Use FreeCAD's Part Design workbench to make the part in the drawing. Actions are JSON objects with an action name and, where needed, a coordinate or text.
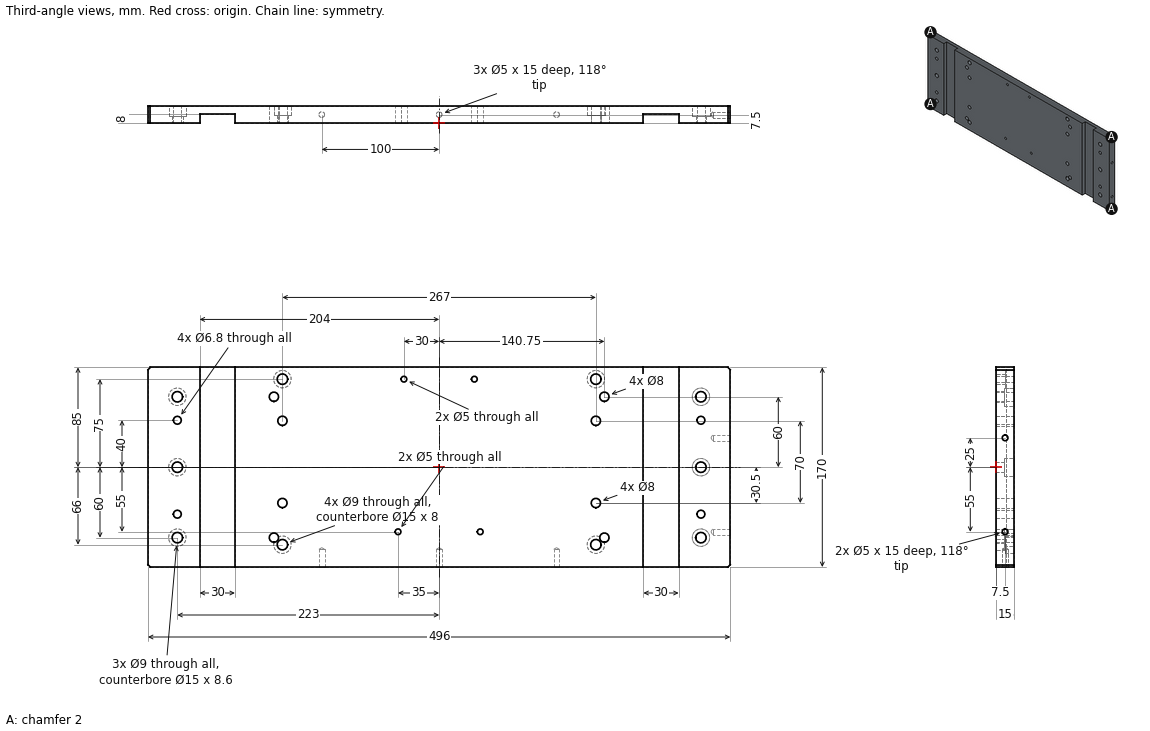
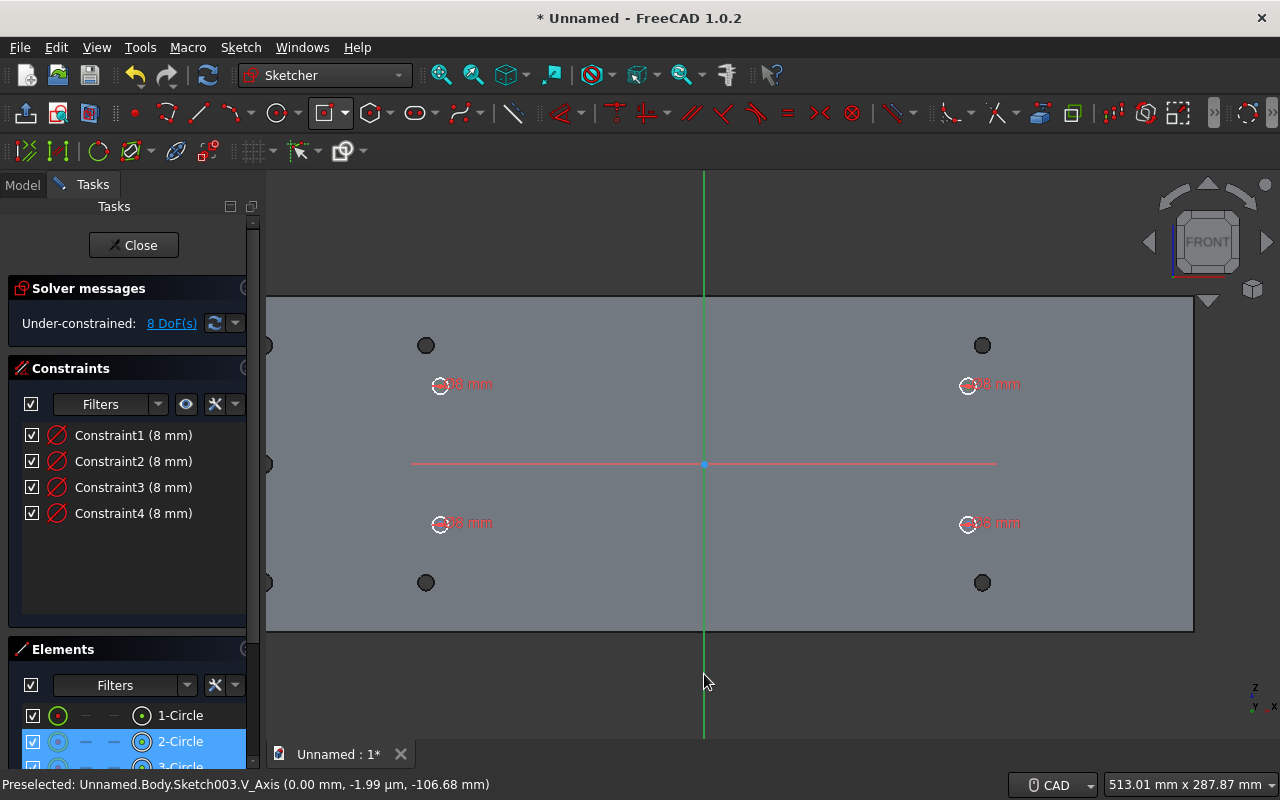
{"action": "left_click", "coordinate": [820, 114]}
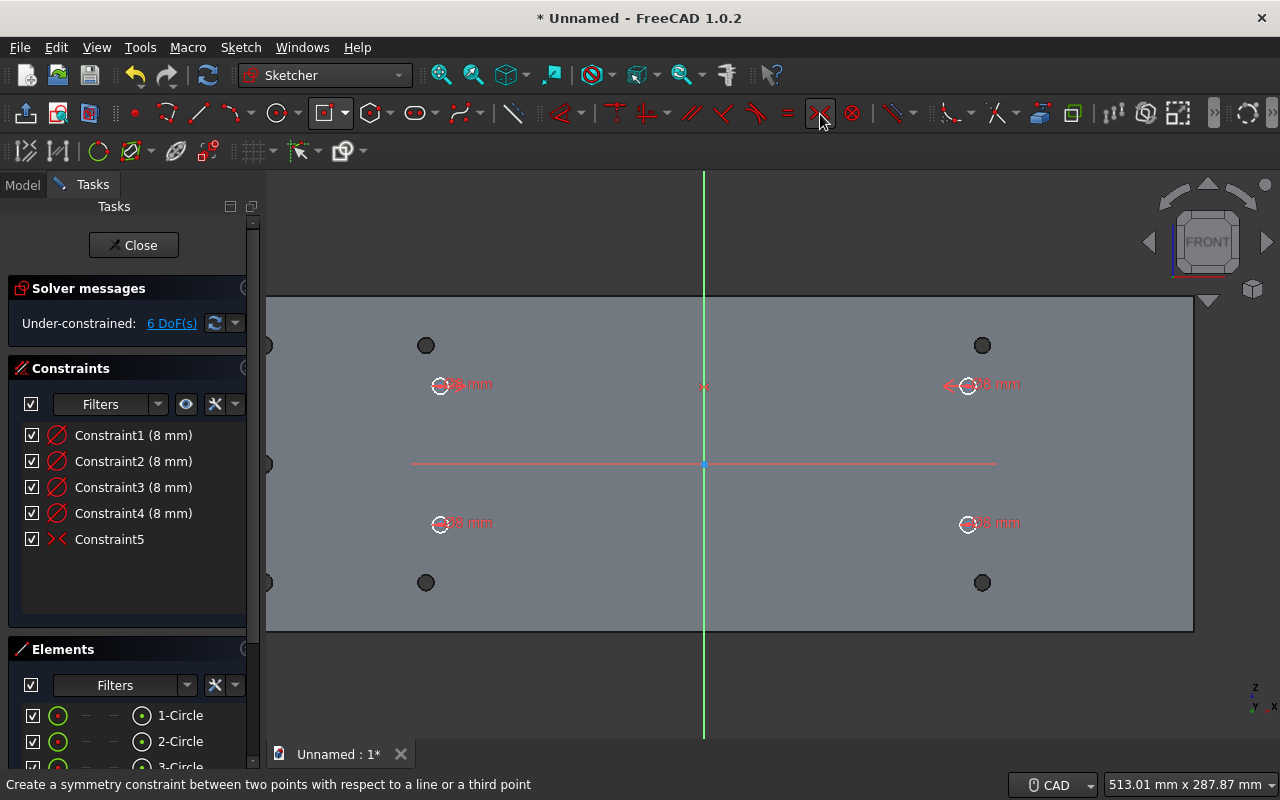
{"action": "left_click", "coordinate": [968, 525]}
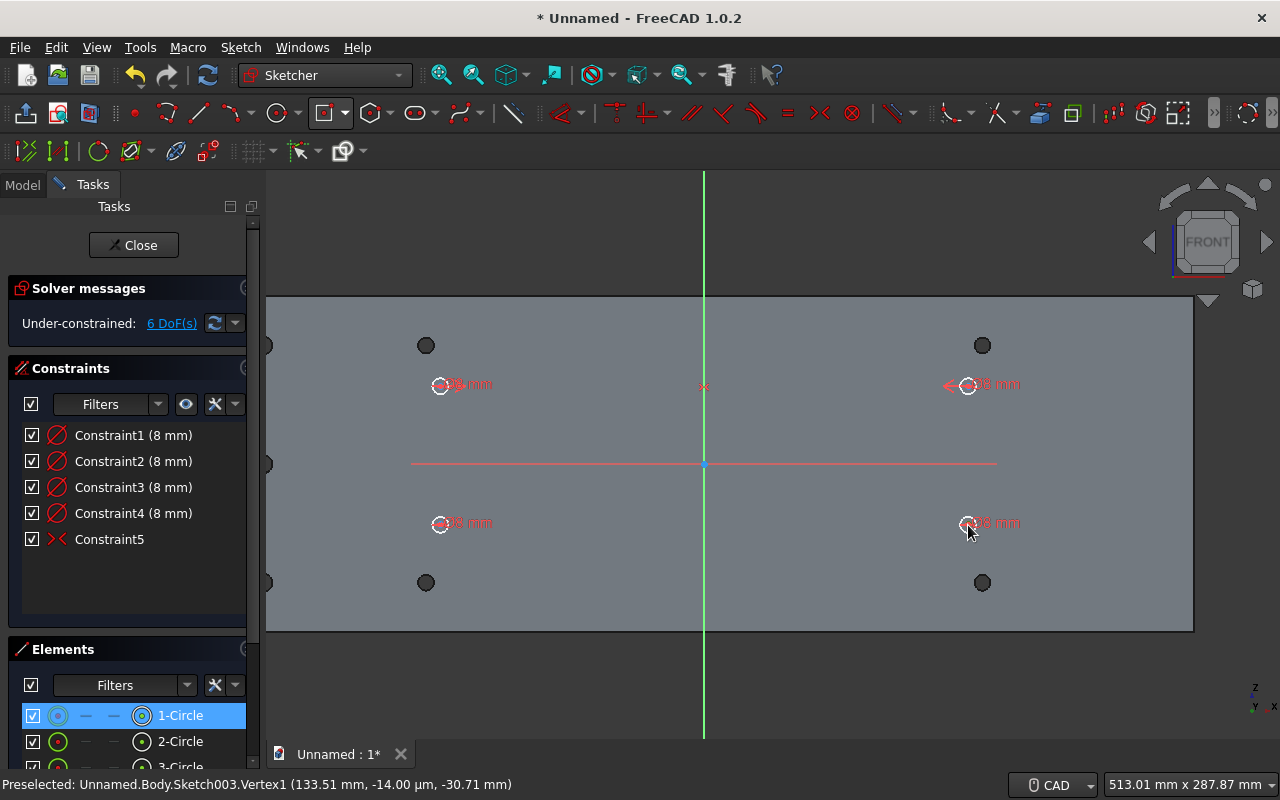
{"action": "left_click", "coordinate": [440, 525]}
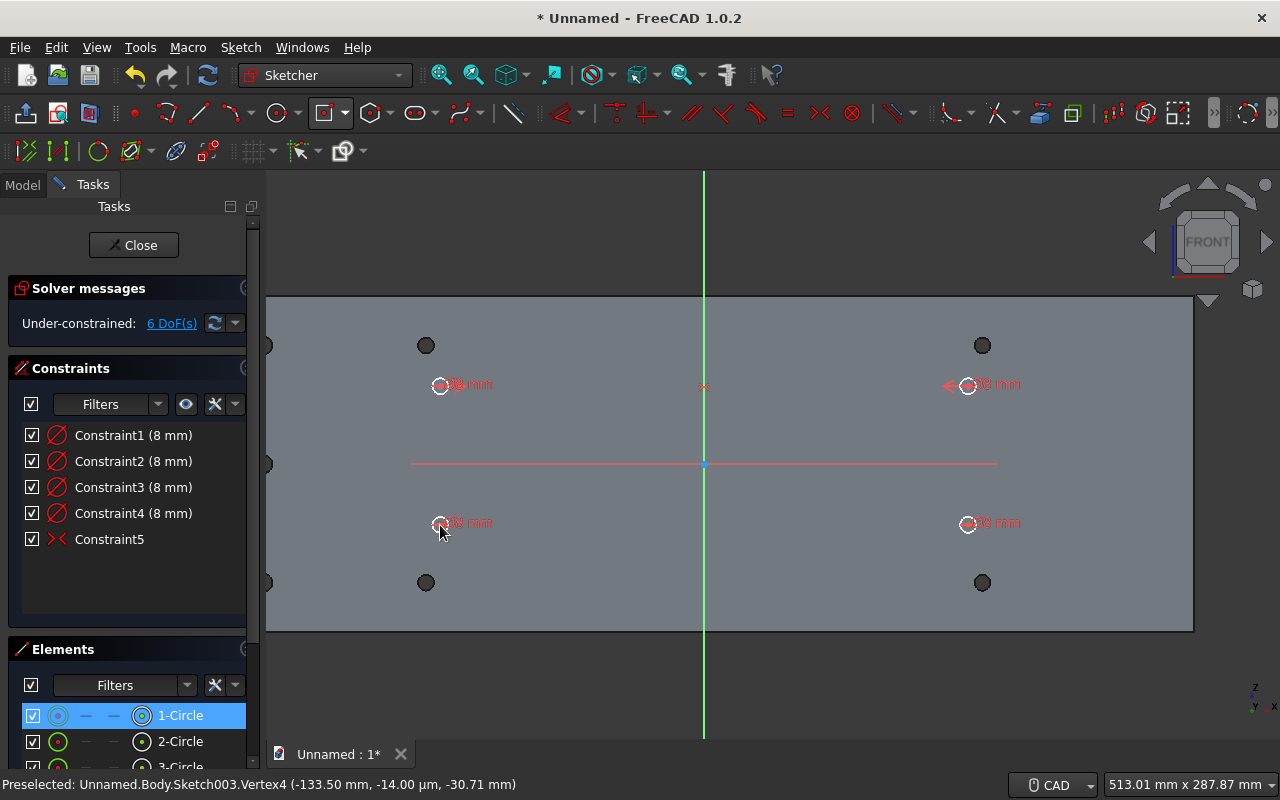
{"action": "left_click", "coordinate": [704, 674]}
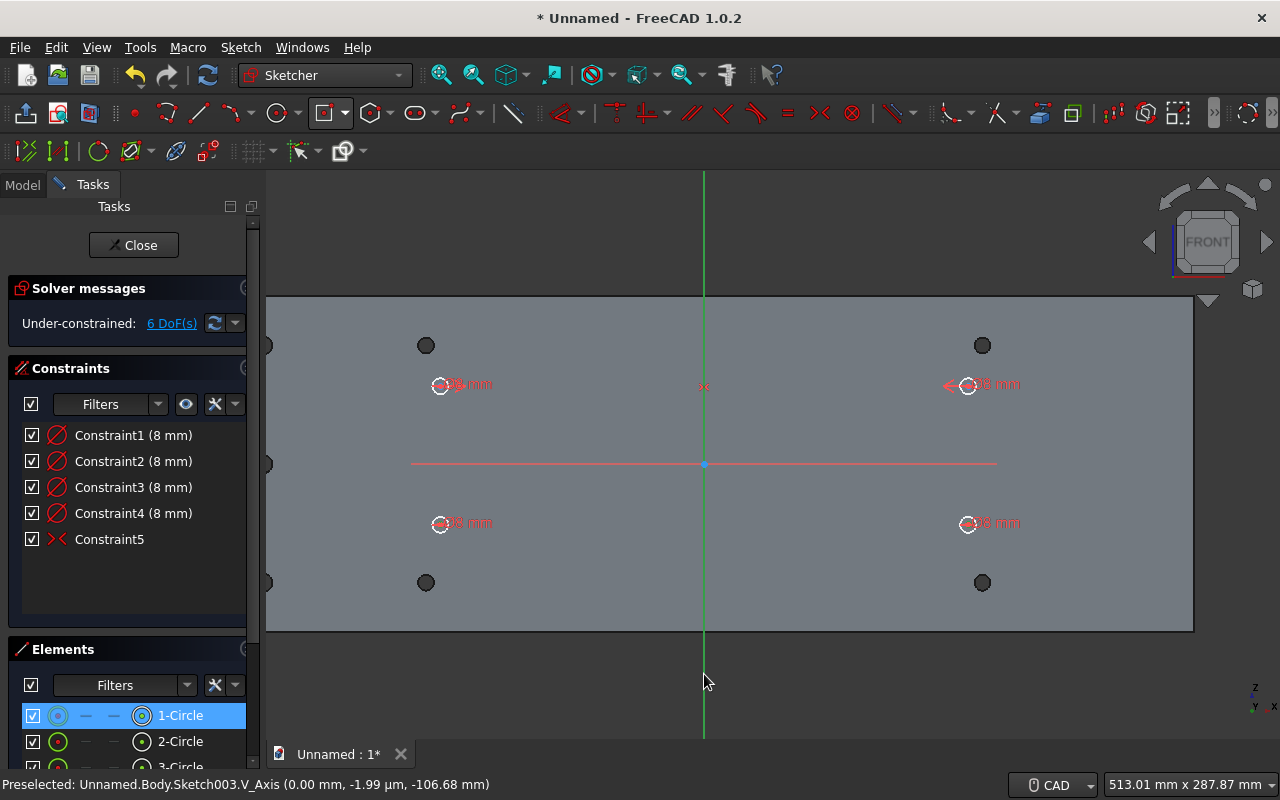
{"action": "left_click", "coordinate": [820, 114]}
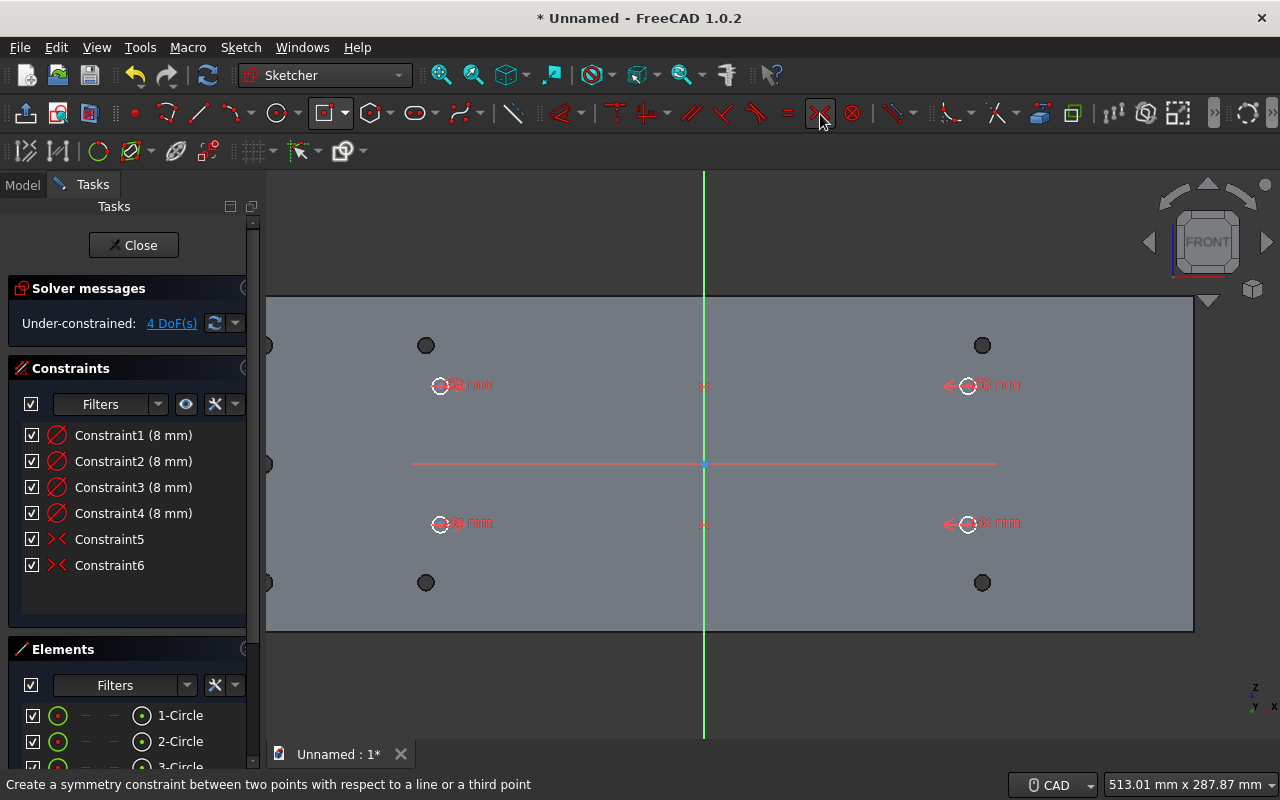
{"action": "left_click", "coordinate": [560, 114]}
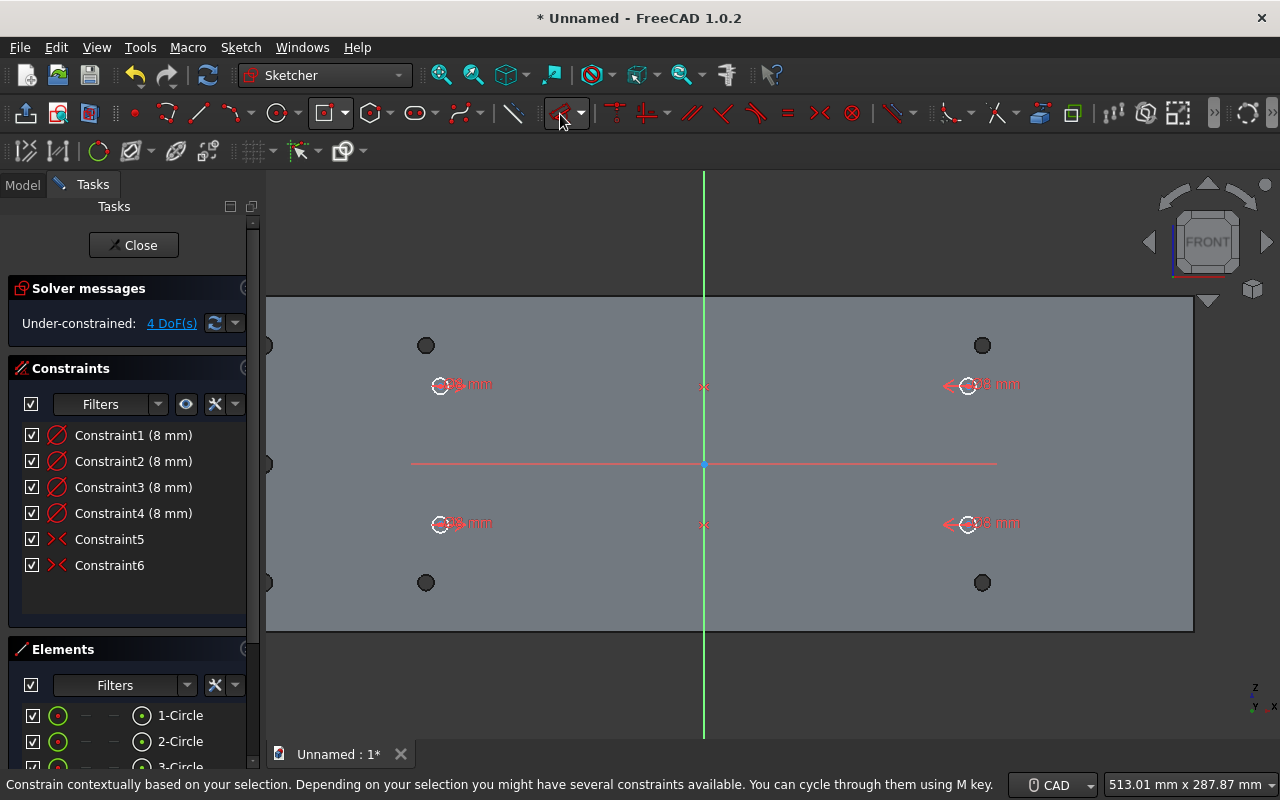
{"action": "left_click", "coordinate": [968, 525]}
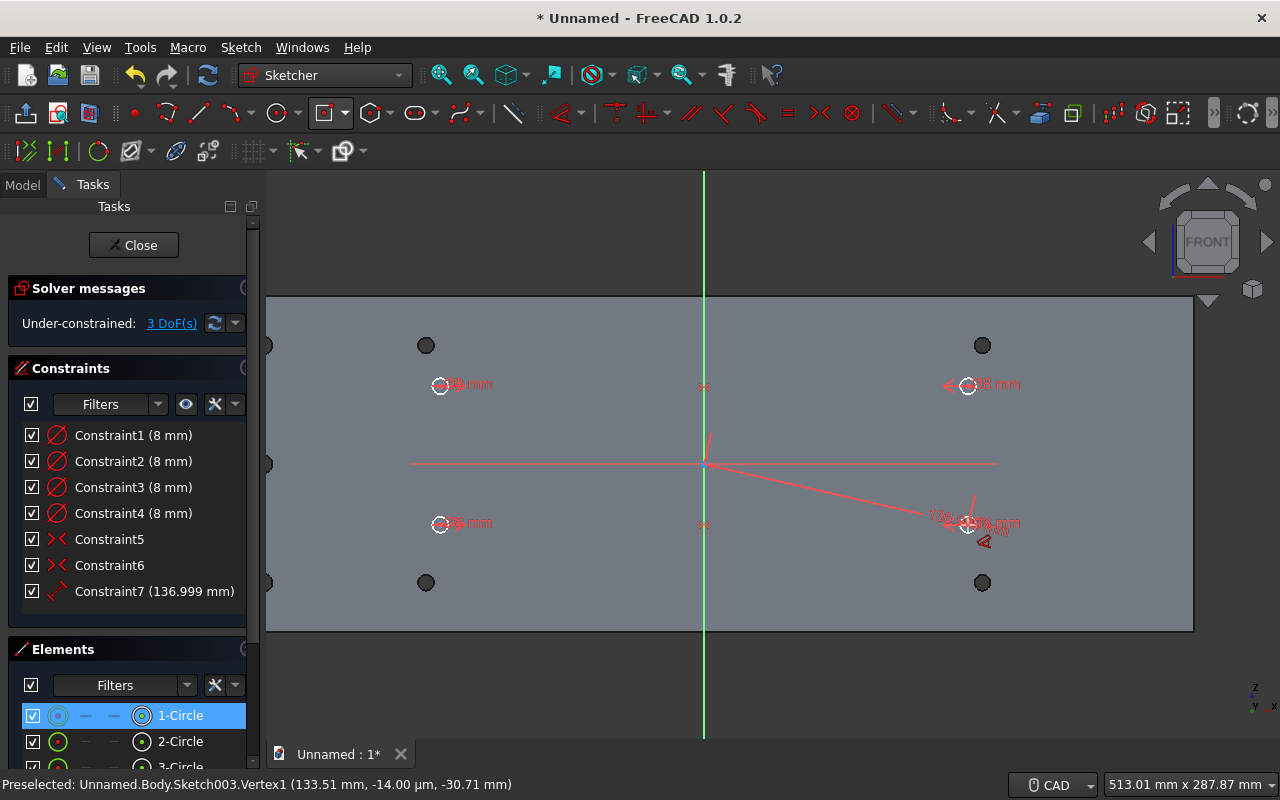
{"action": "left_click", "coordinate": [968, 386]}
{"action": "left_click", "coordinate": [1002, 424]}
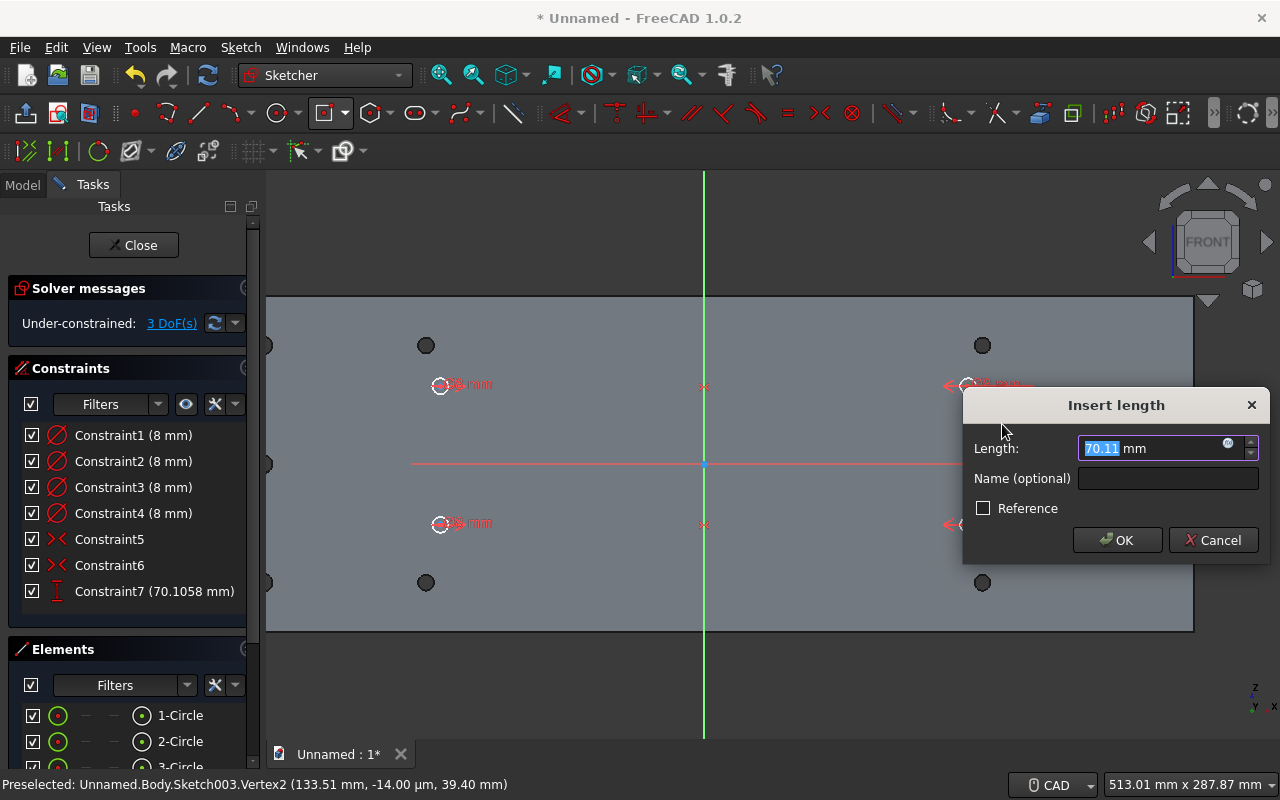
{"action": "type", "text": "70"}
{"action": "key", "text": "Return"}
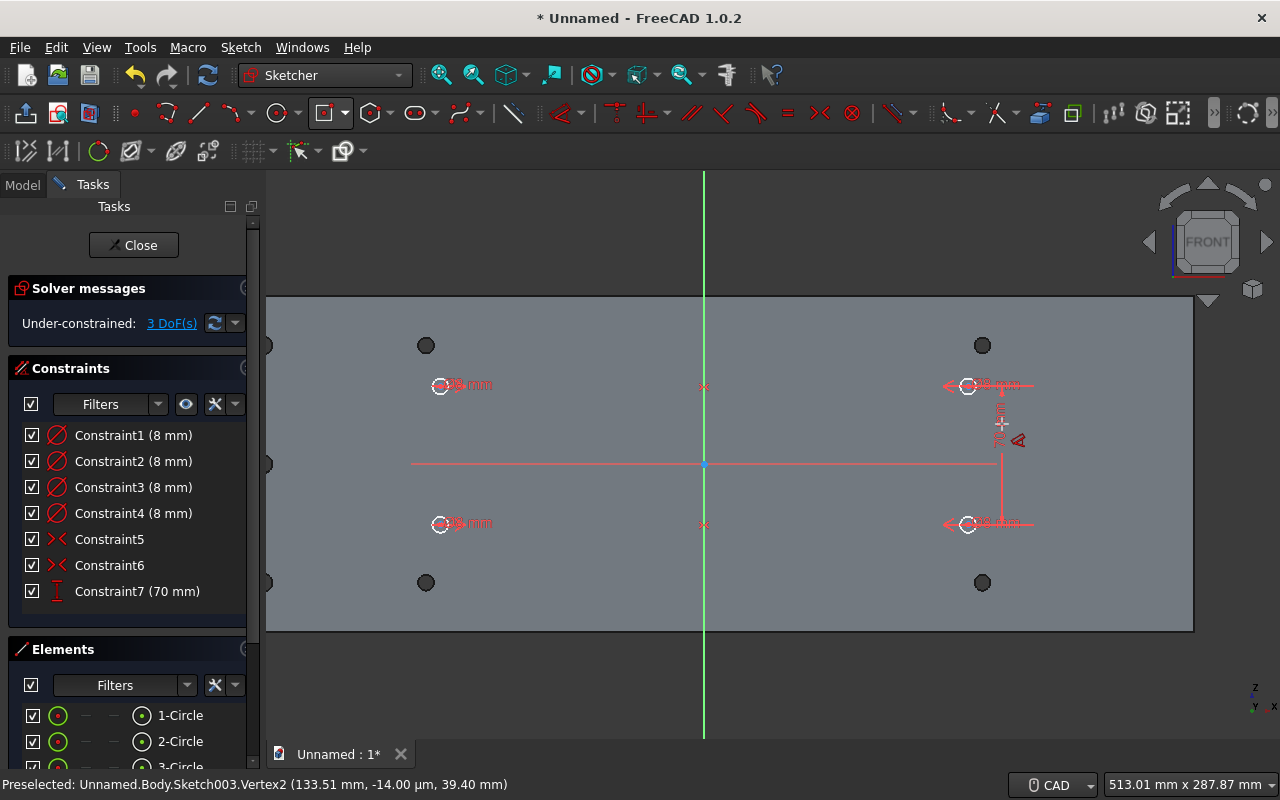
{"action": "left_click", "coordinate": [968, 525]}
{"action": "left_click", "coordinate": [1002, 494]}